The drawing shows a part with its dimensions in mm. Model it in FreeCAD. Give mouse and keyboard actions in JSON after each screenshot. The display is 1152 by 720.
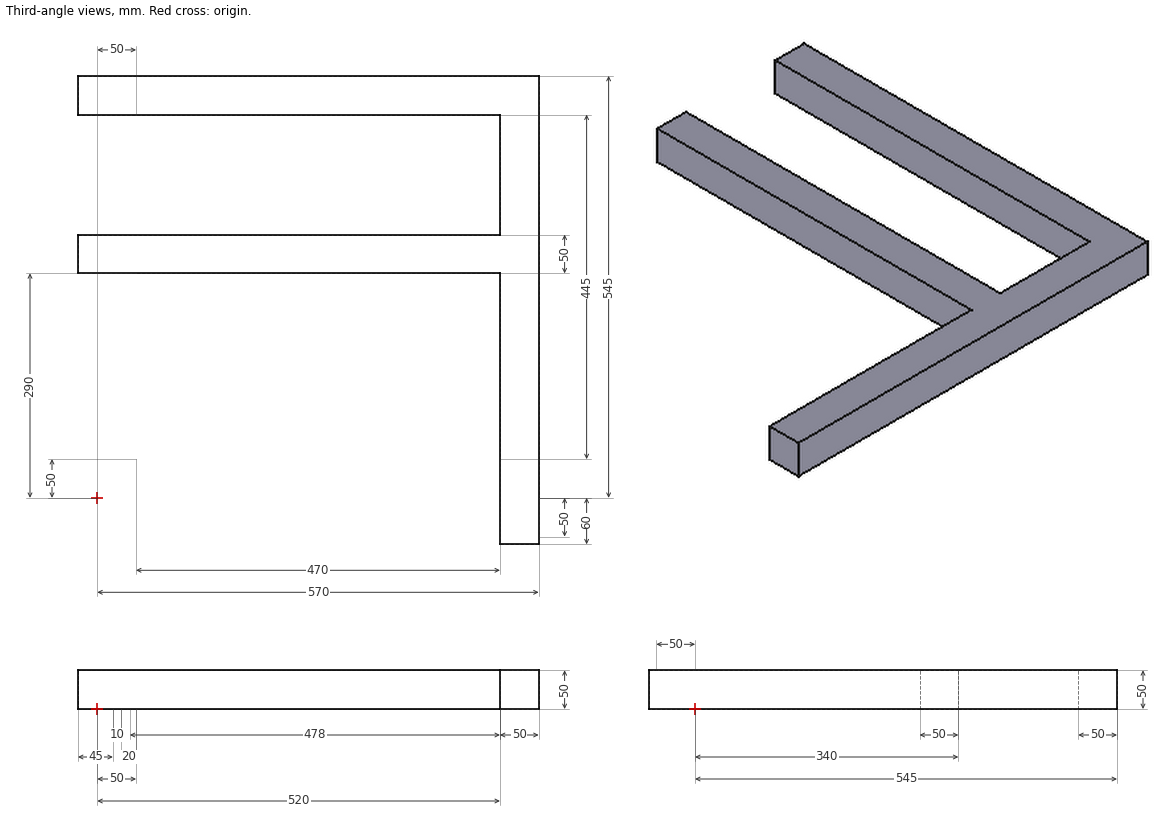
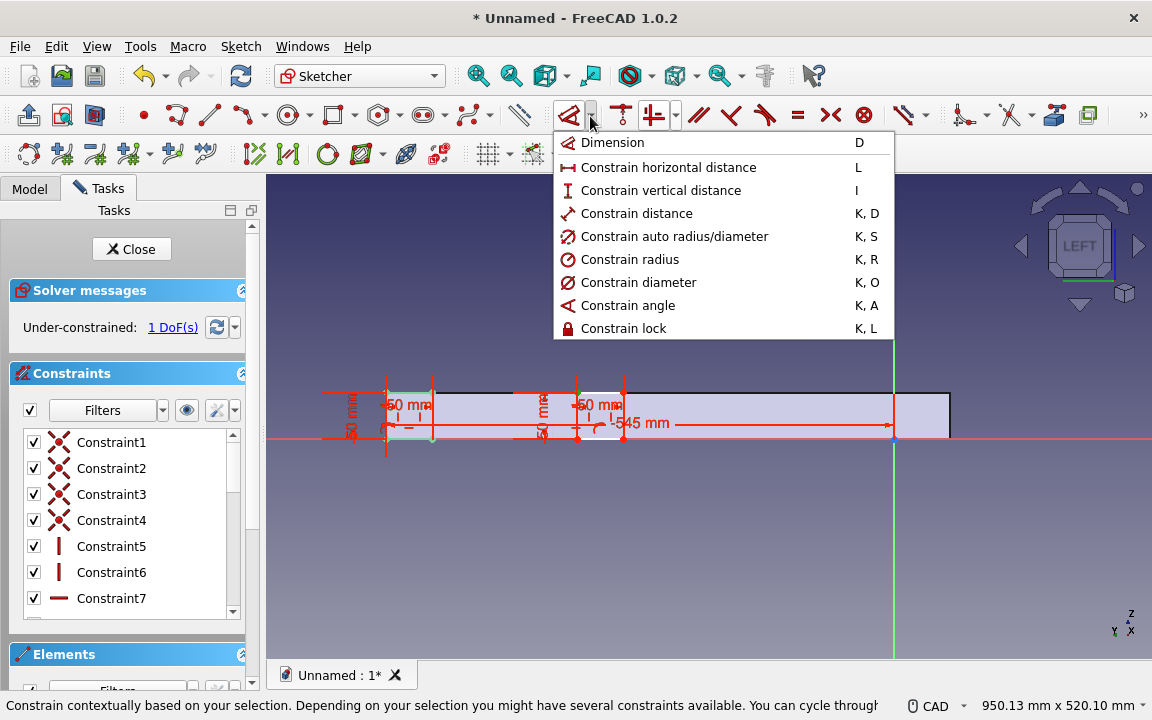
{"action": "left_click", "coordinate": [724, 168]}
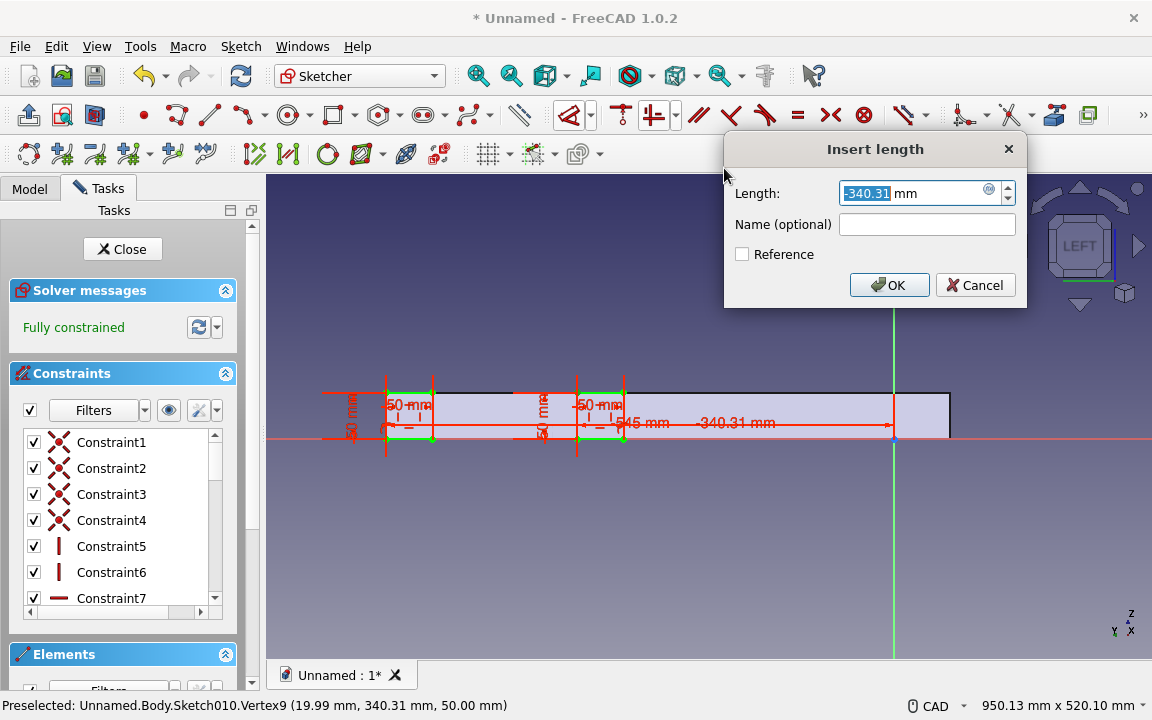
{"action": "type", "text": "-340"}
{"action": "key", "text": "Return"}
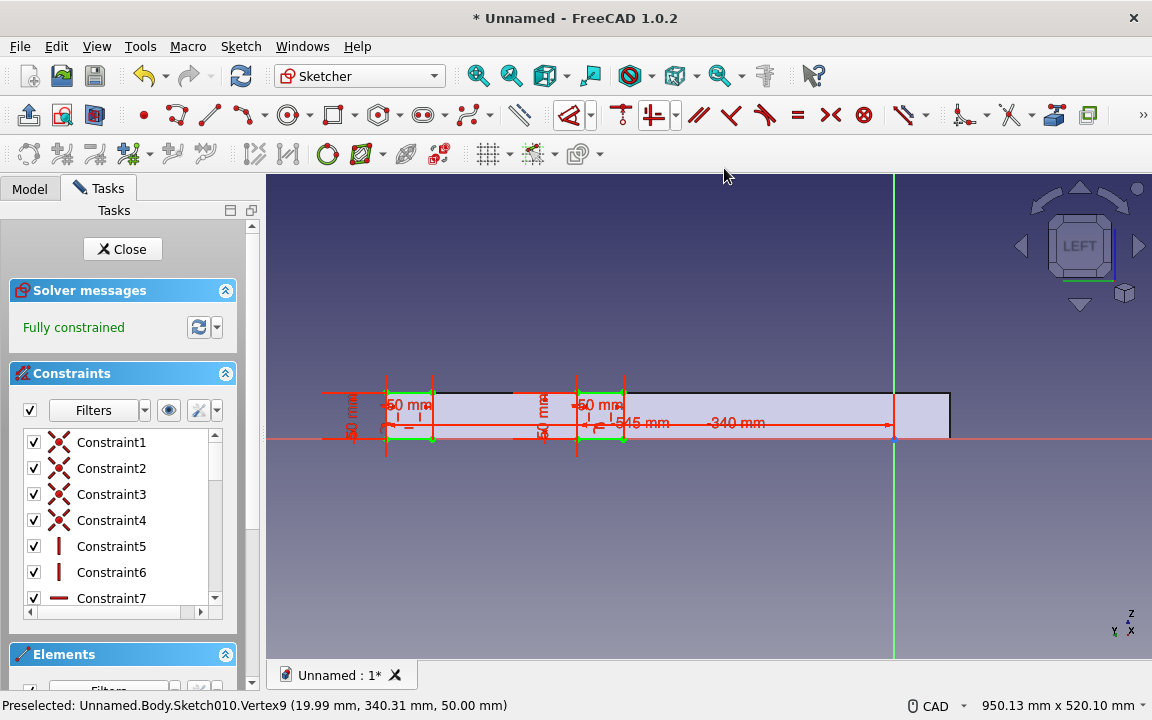
{"action": "left_click", "coordinate": [123, 249]}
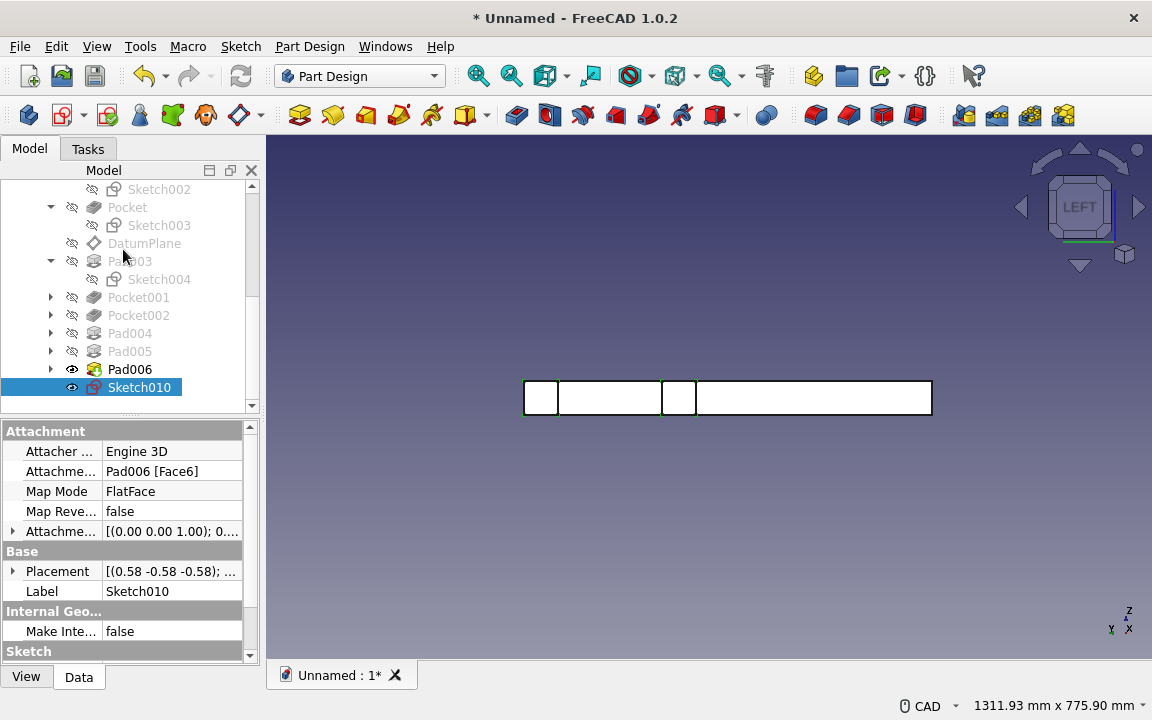
{"action": "left_click", "coordinate": [300, 116]}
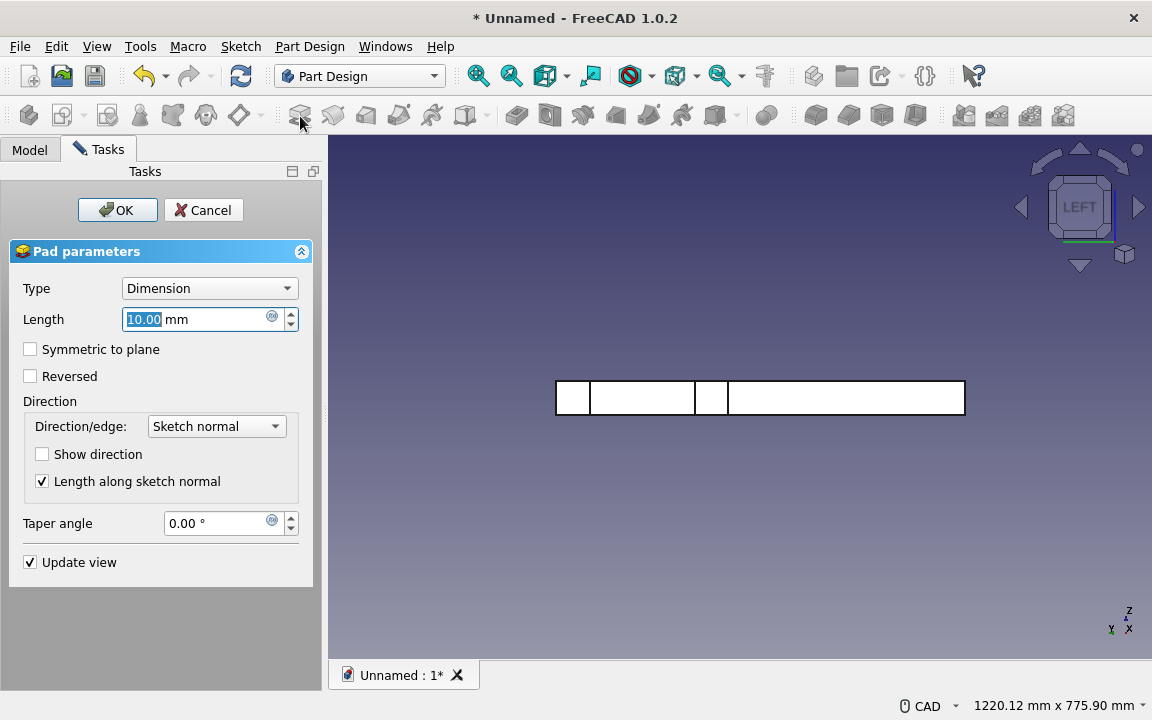
{"action": "type", "text": "45"}
{"action": "key", "text": "Tab"}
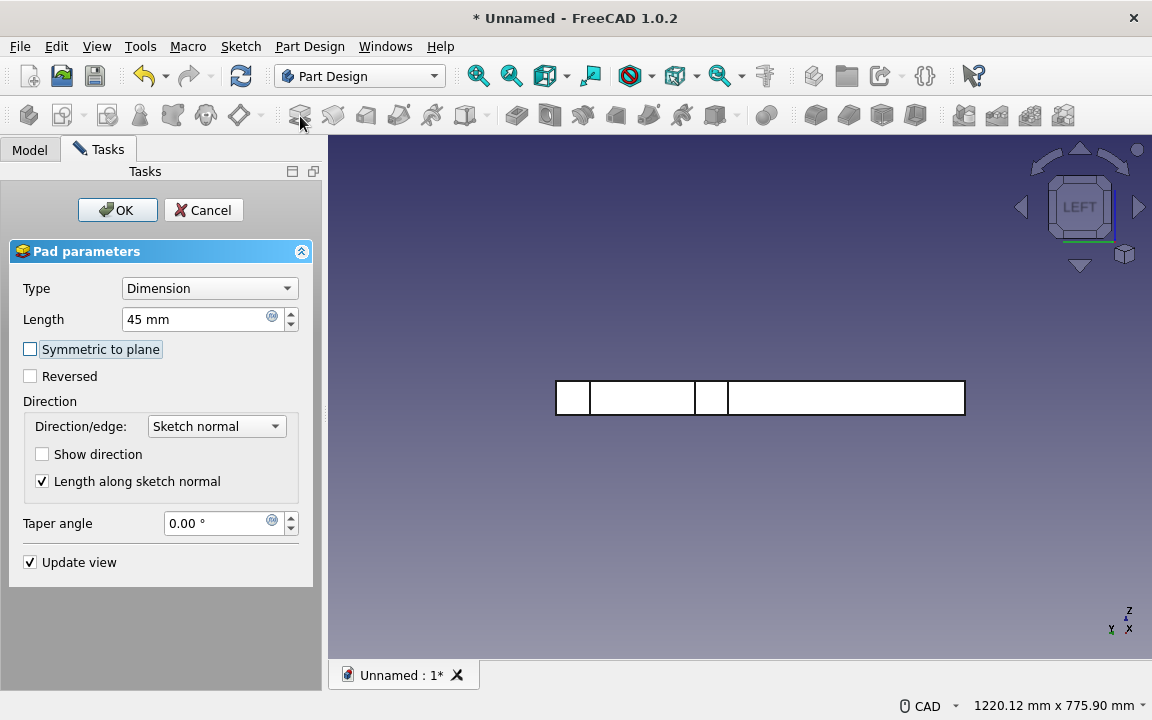
{"action": "left_click", "coordinate": [118, 210]}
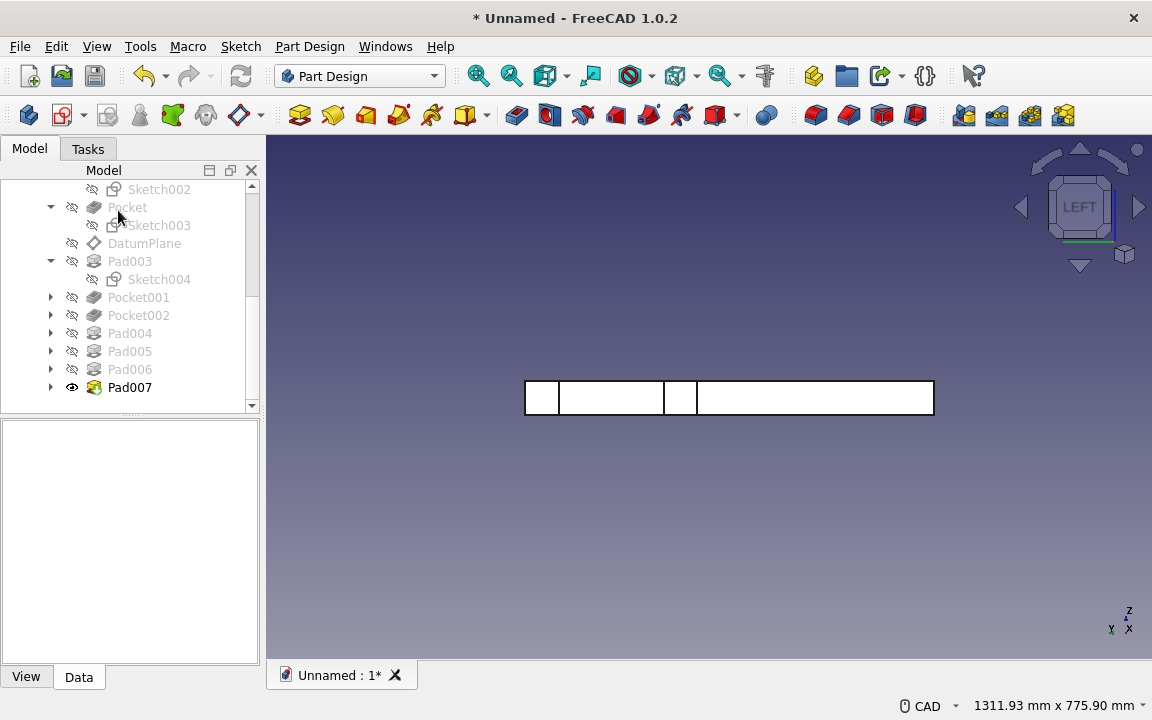
{"action": "key", "text": "0"}